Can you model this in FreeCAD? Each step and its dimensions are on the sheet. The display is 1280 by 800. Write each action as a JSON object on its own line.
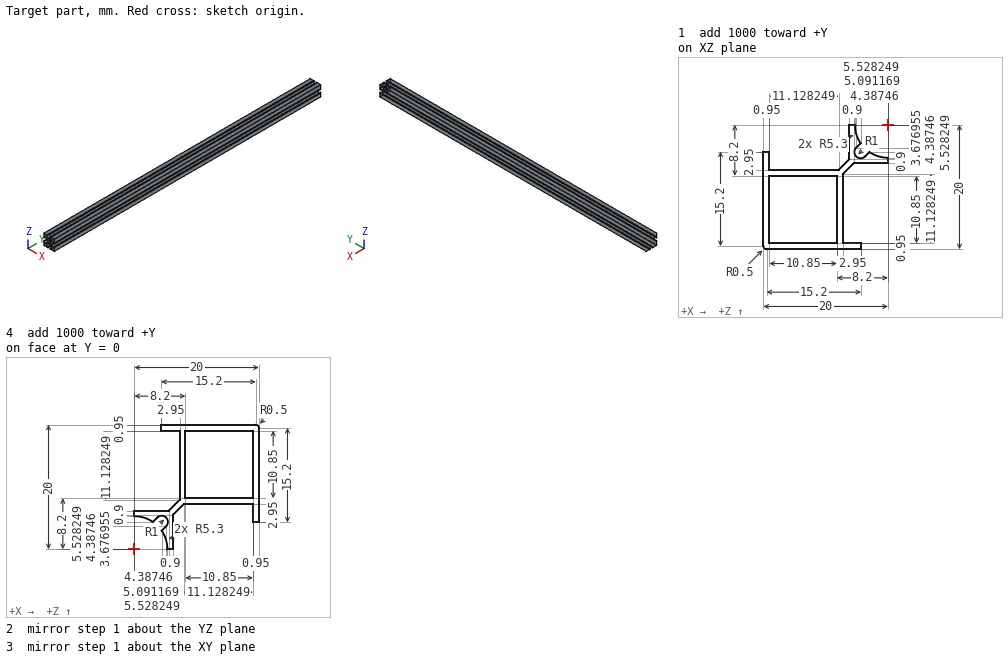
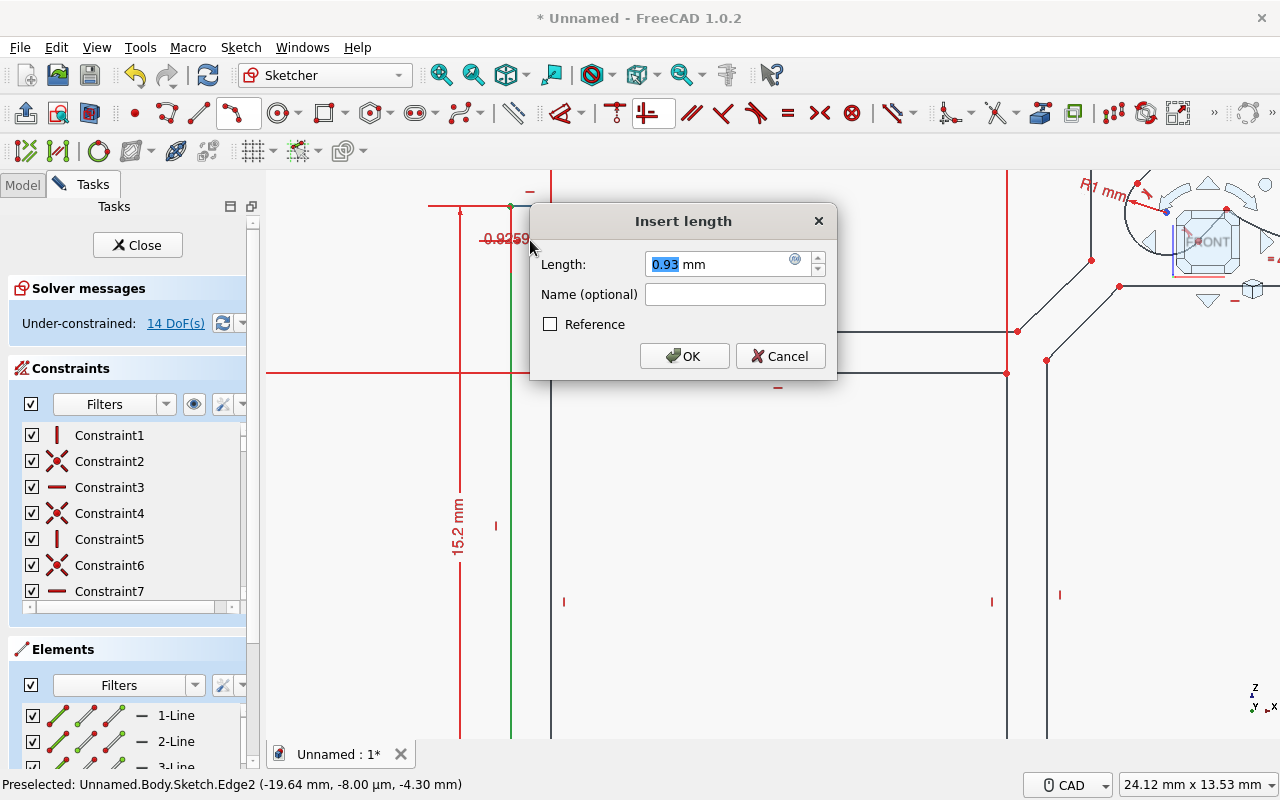
{"action": "type", "text": "0.95"}
{"action": "key", "text": "Return"}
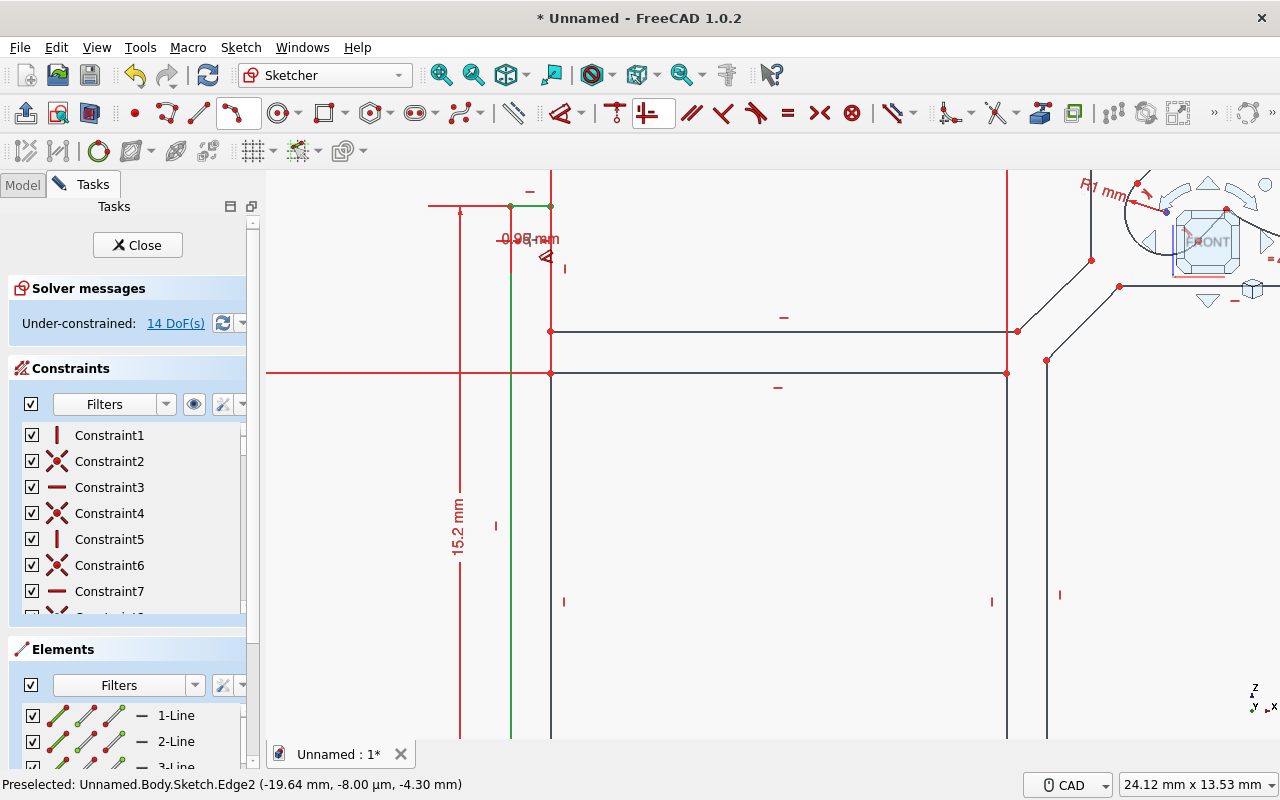
{"action": "left_click", "coordinate": [551, 244]}
{"action": "left_click", "coordinate": [585, 269]}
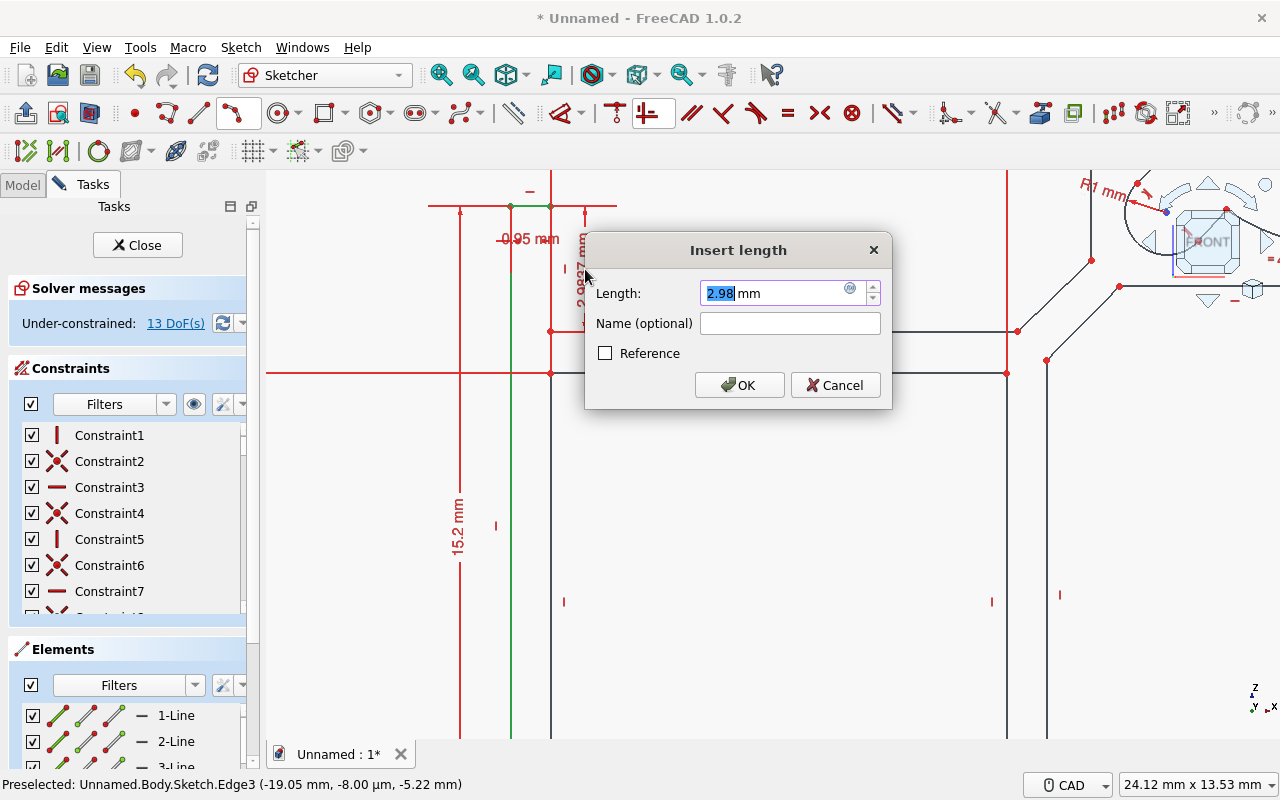
{"action": "type", "text": "2.95"}
{"action": "key", "text": "Return"}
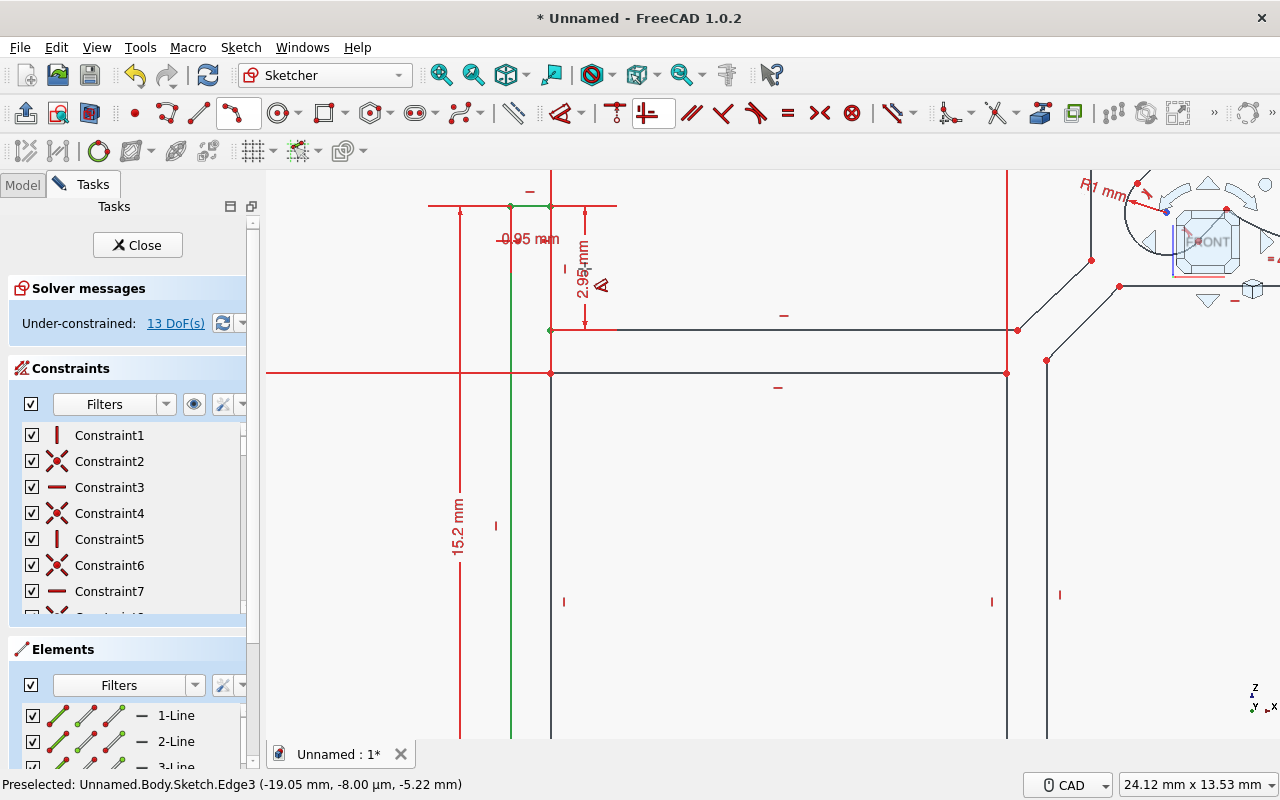
{"action": "scroll", "coordinate": [519, 462], "scroll_direction": "down", "scroll_amount": 4}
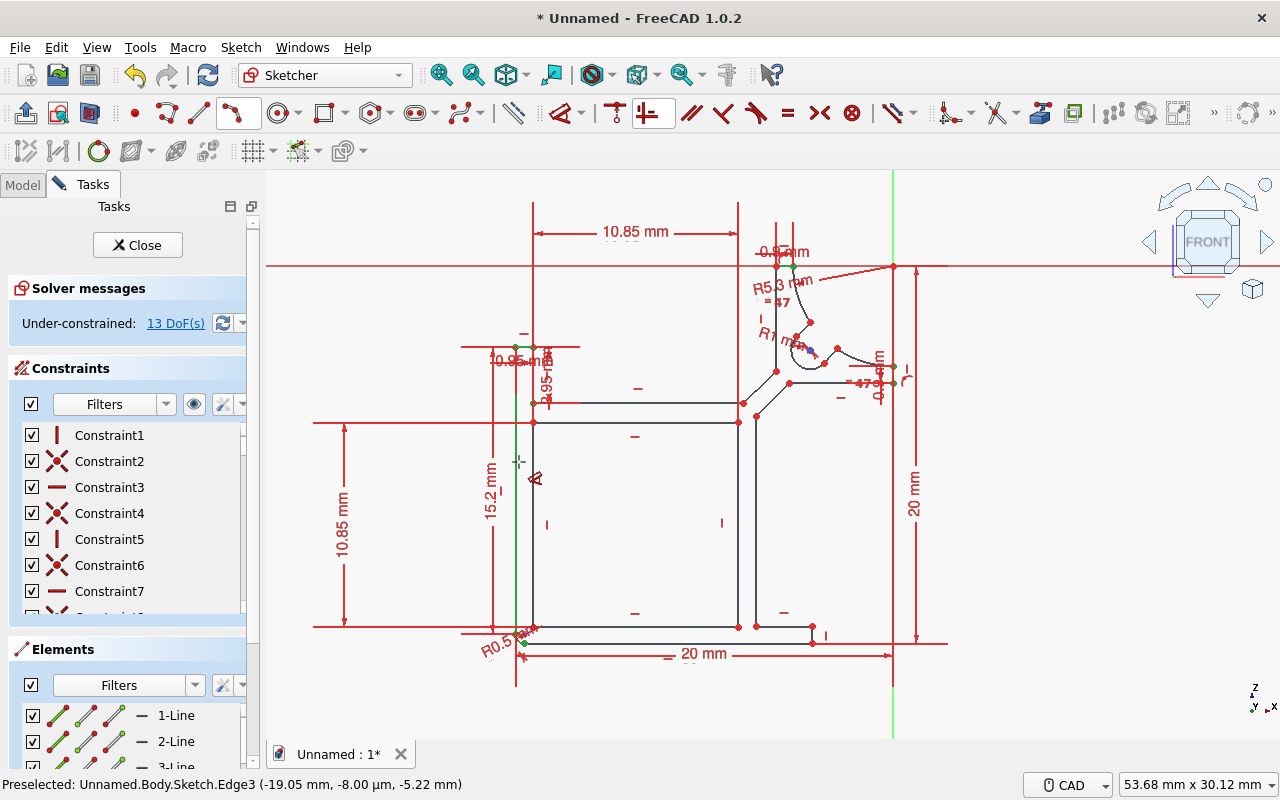
{"action": "left_click", "coordinate": [773, 627]}
{"action": "left_click", "coordinate": [784, 661]}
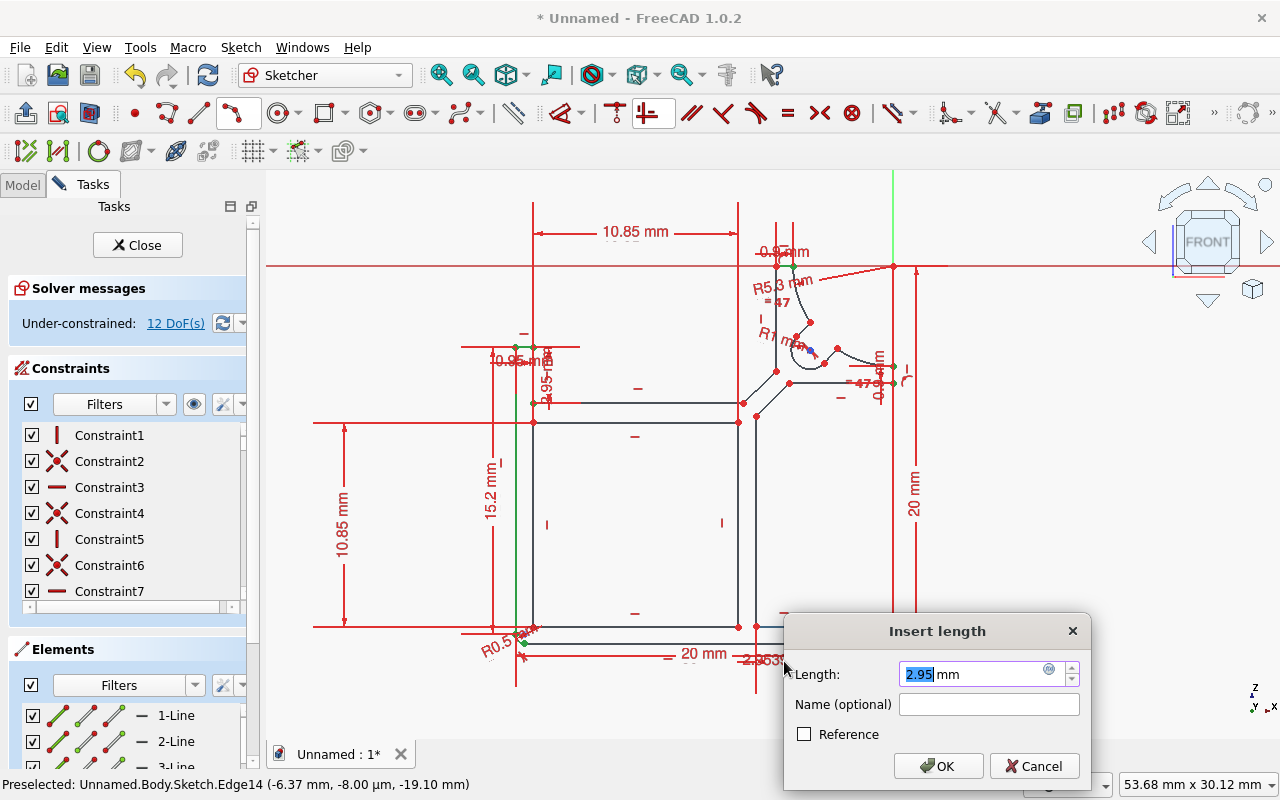
{"action": "type", "text": "2.95"}
{"action": "key", "text": "Return"}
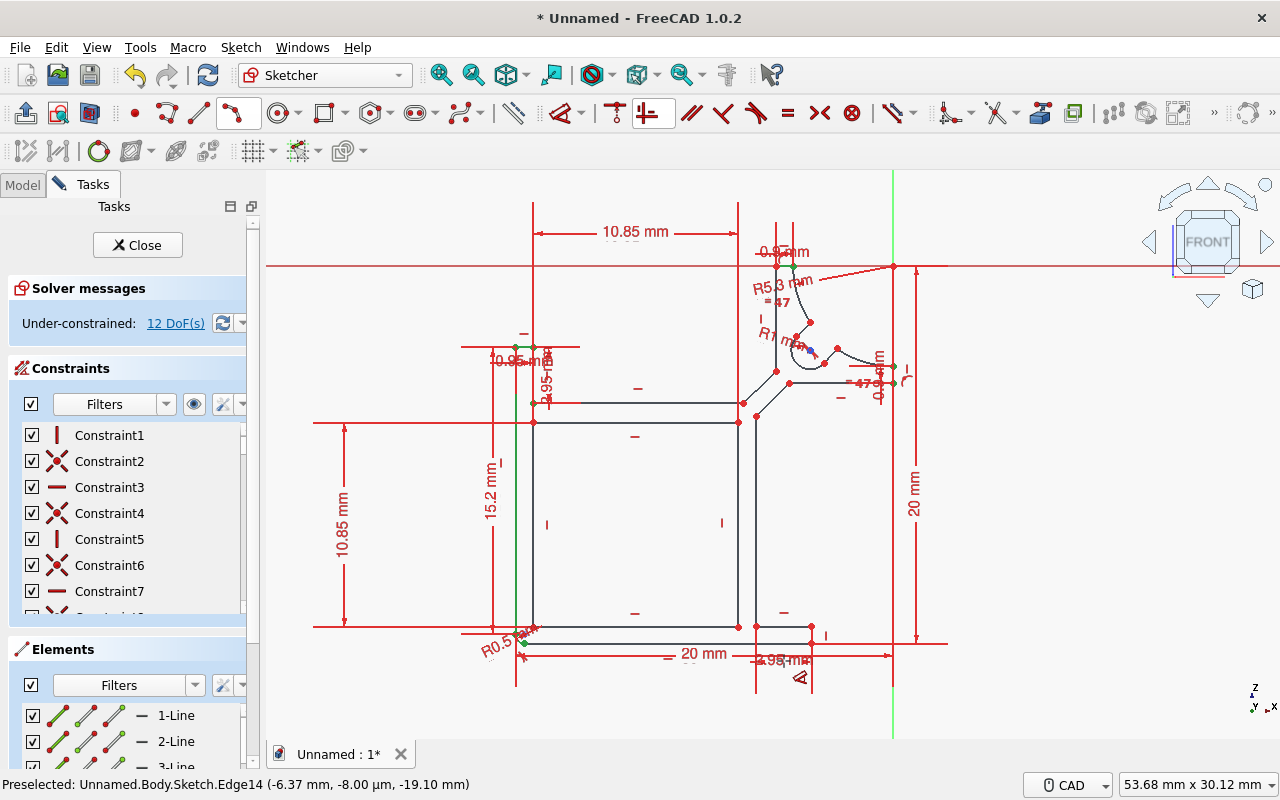
{"action": "scroll", "coordinate": [812, 635], "scroll_direction": "up", "scroll_amount": 4}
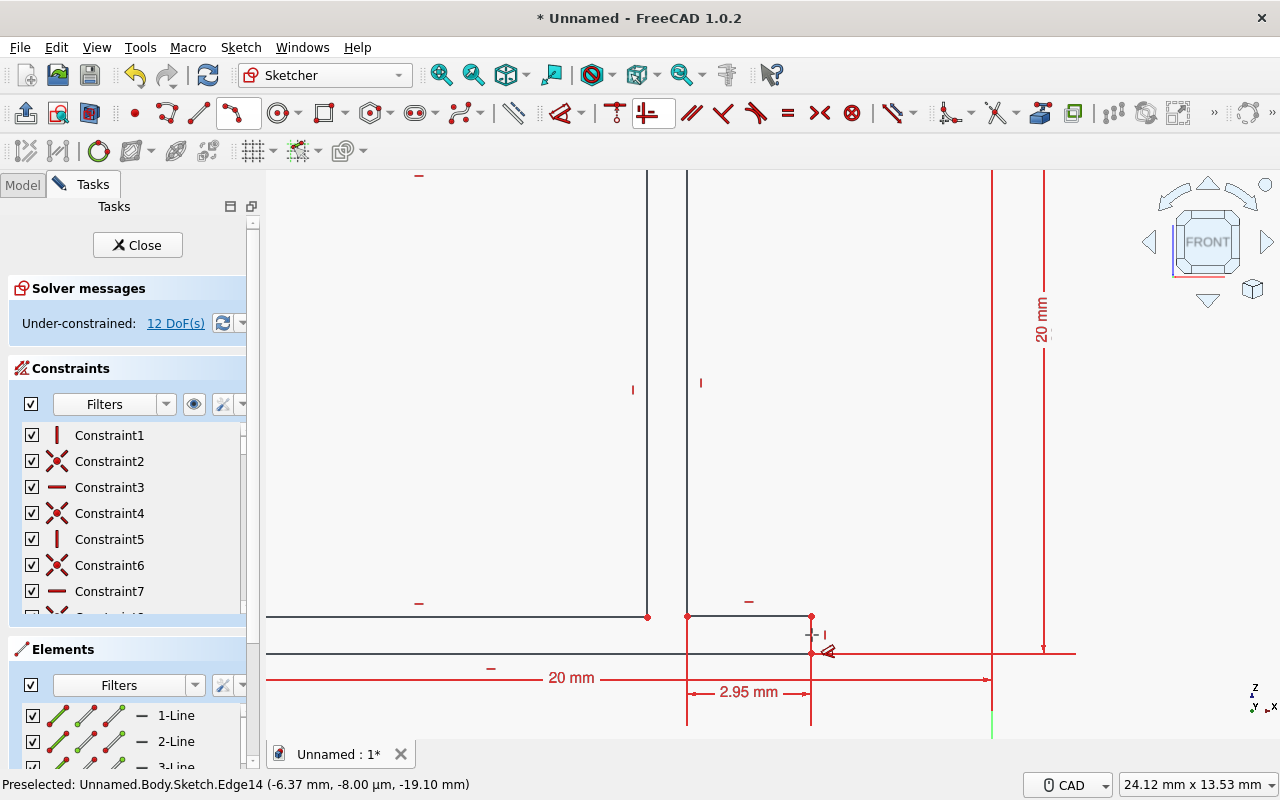
{"action": "left_click", "coordinate": [811, 635]}
{"action": "left_click", "coordinate": [845, 635]}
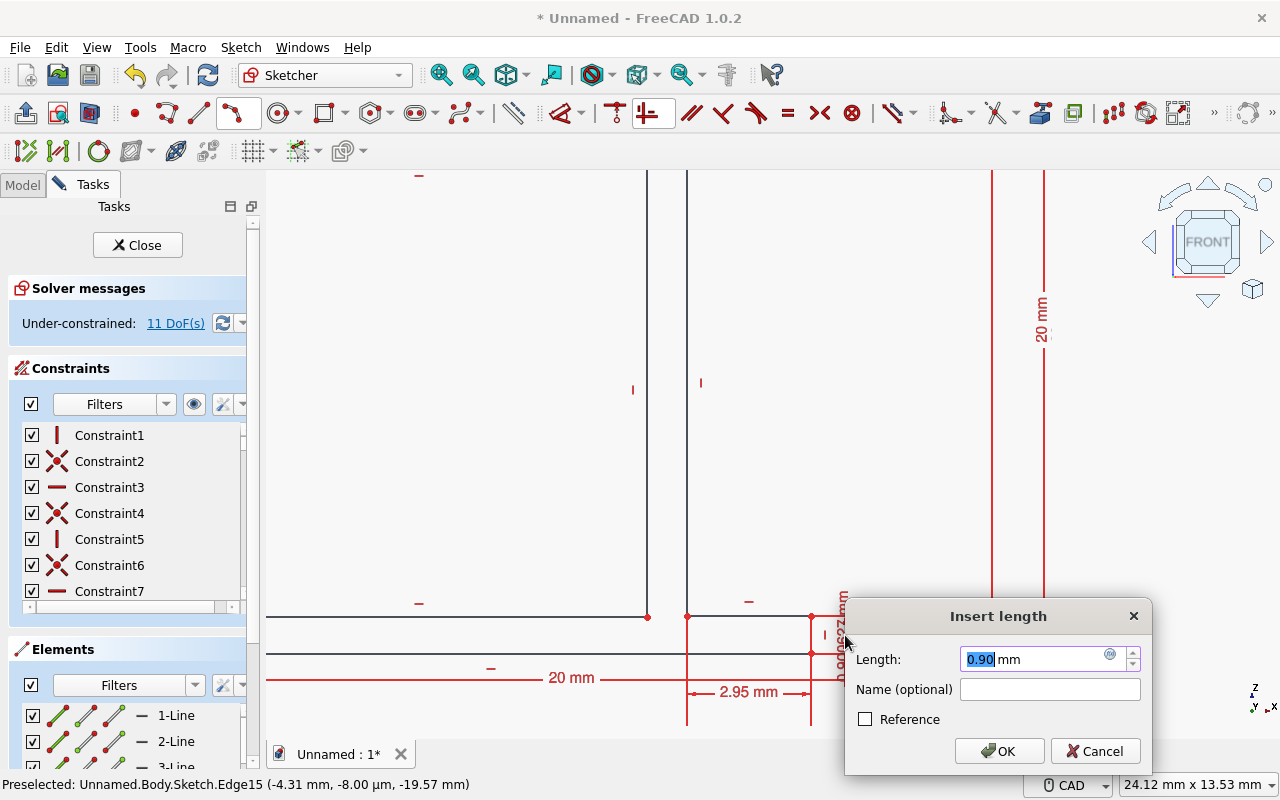
{"action": "type", "text": "0.95"}
{"action": "key", "text": "Return"}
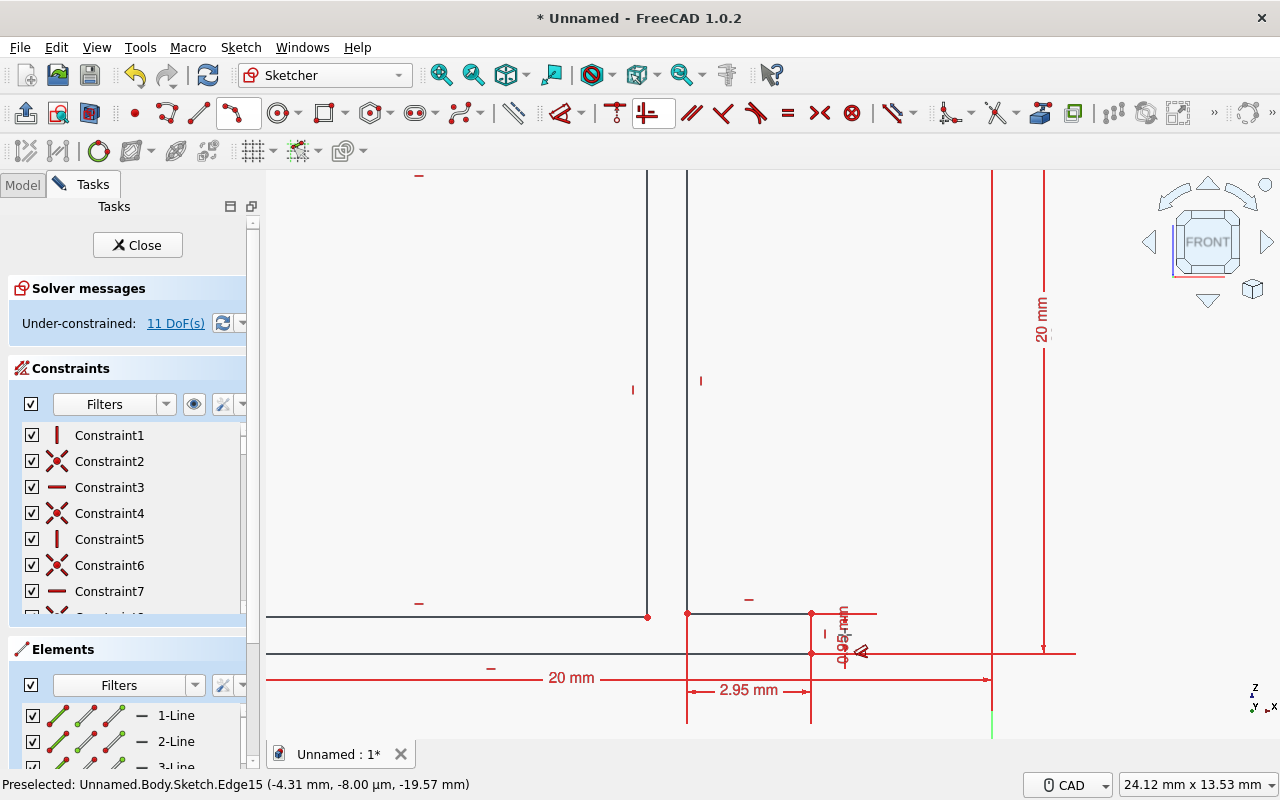
{"action": "left_click", "coordinate": [620, 654]}
{"action": "left_click", "coordinate": [434, 688]}